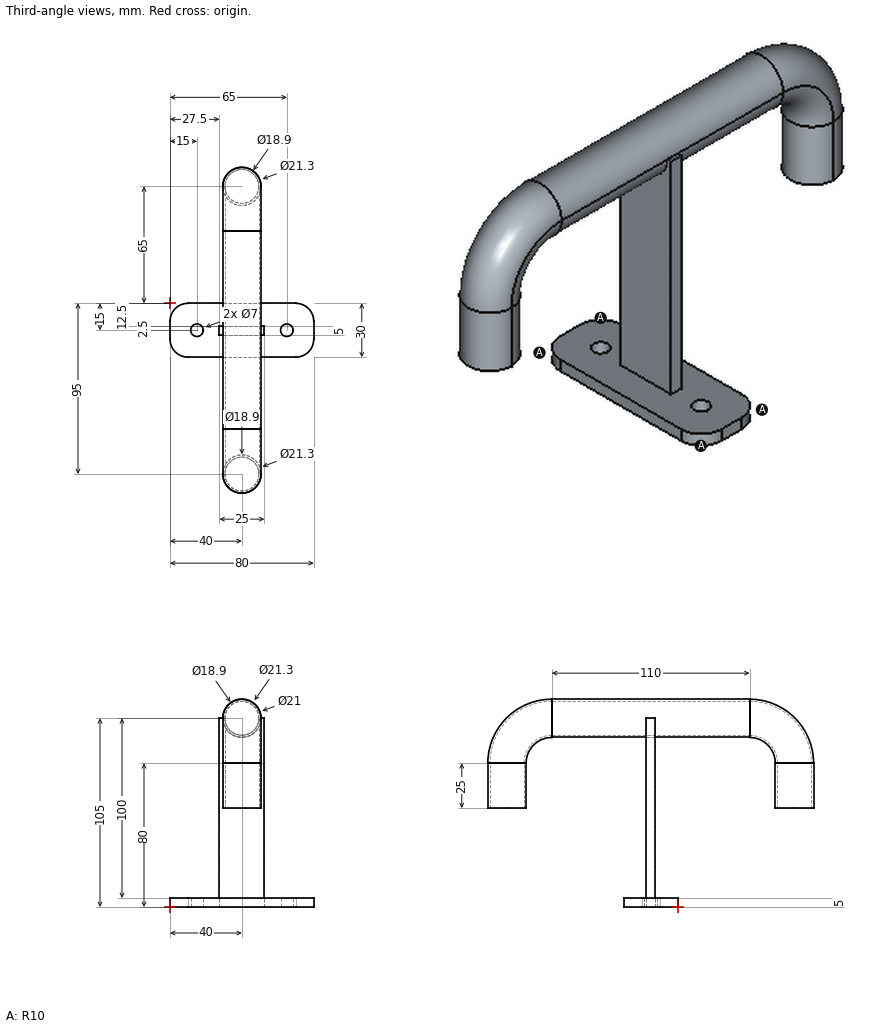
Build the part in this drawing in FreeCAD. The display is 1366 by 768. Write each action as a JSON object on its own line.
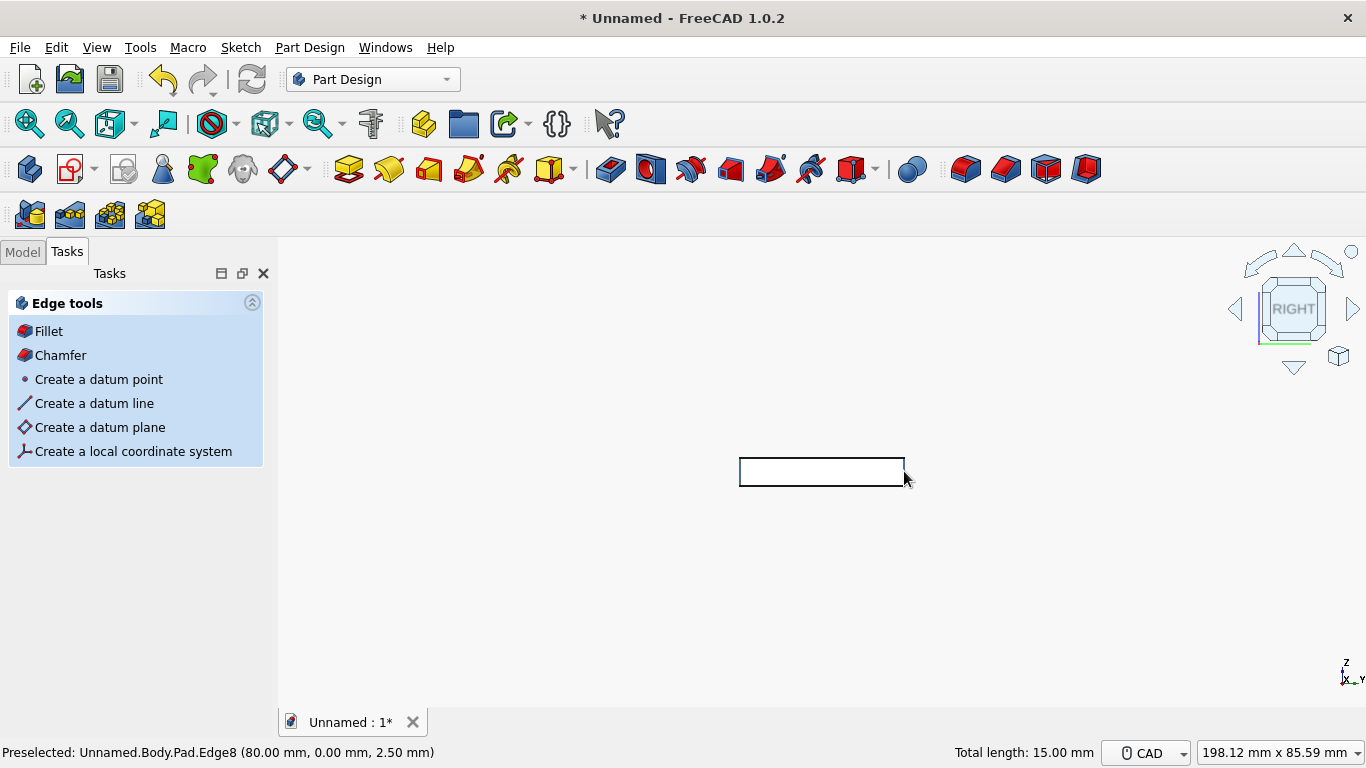
{"action": "key", "text": "5"}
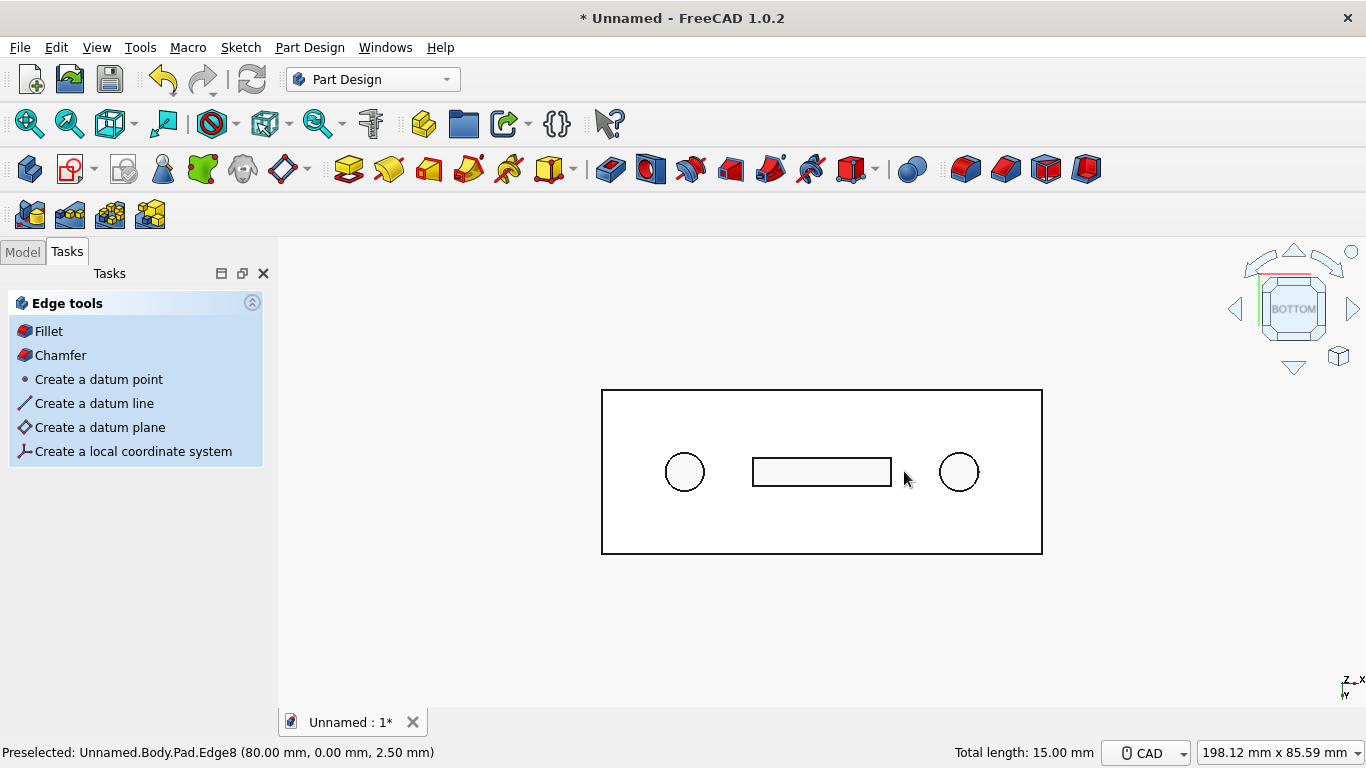
{"action": "left_click", "coordinate": [30, 124]}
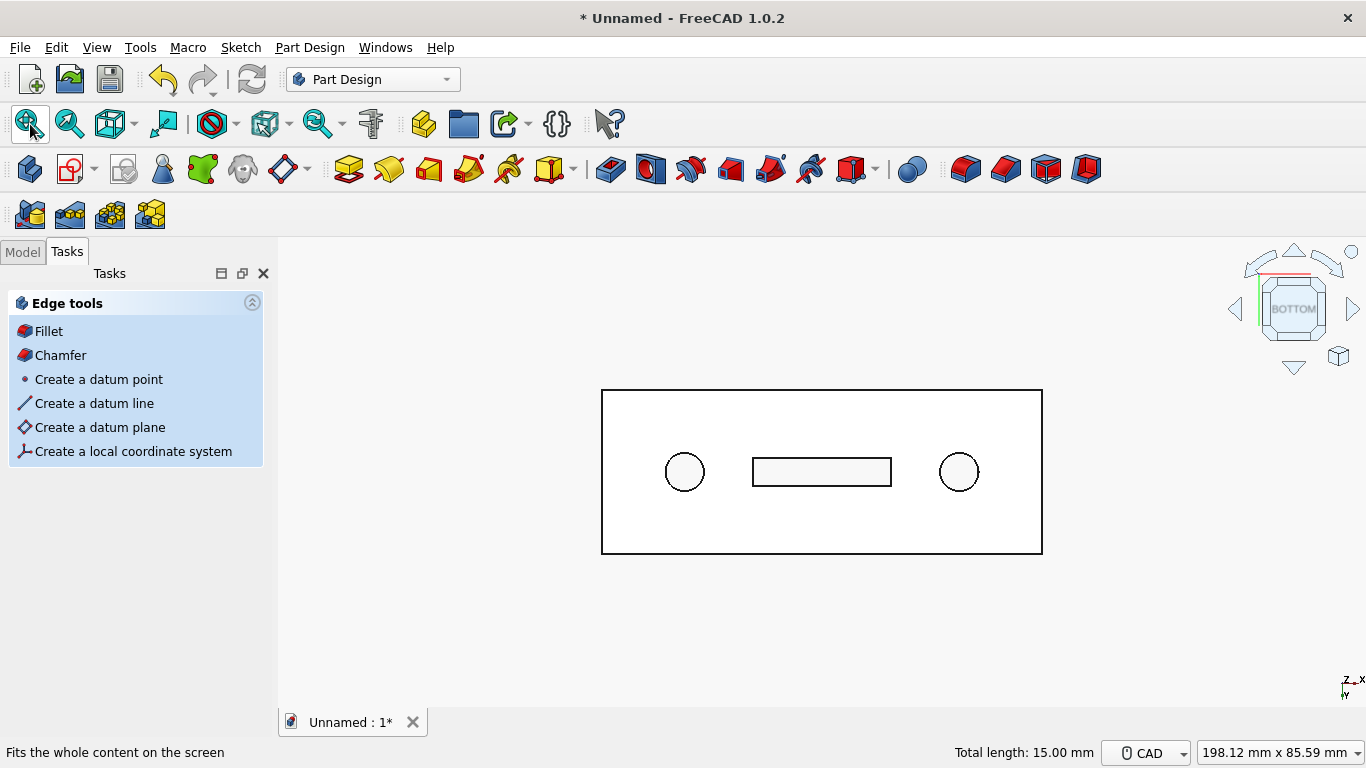
{"action": "key", "text": "4"}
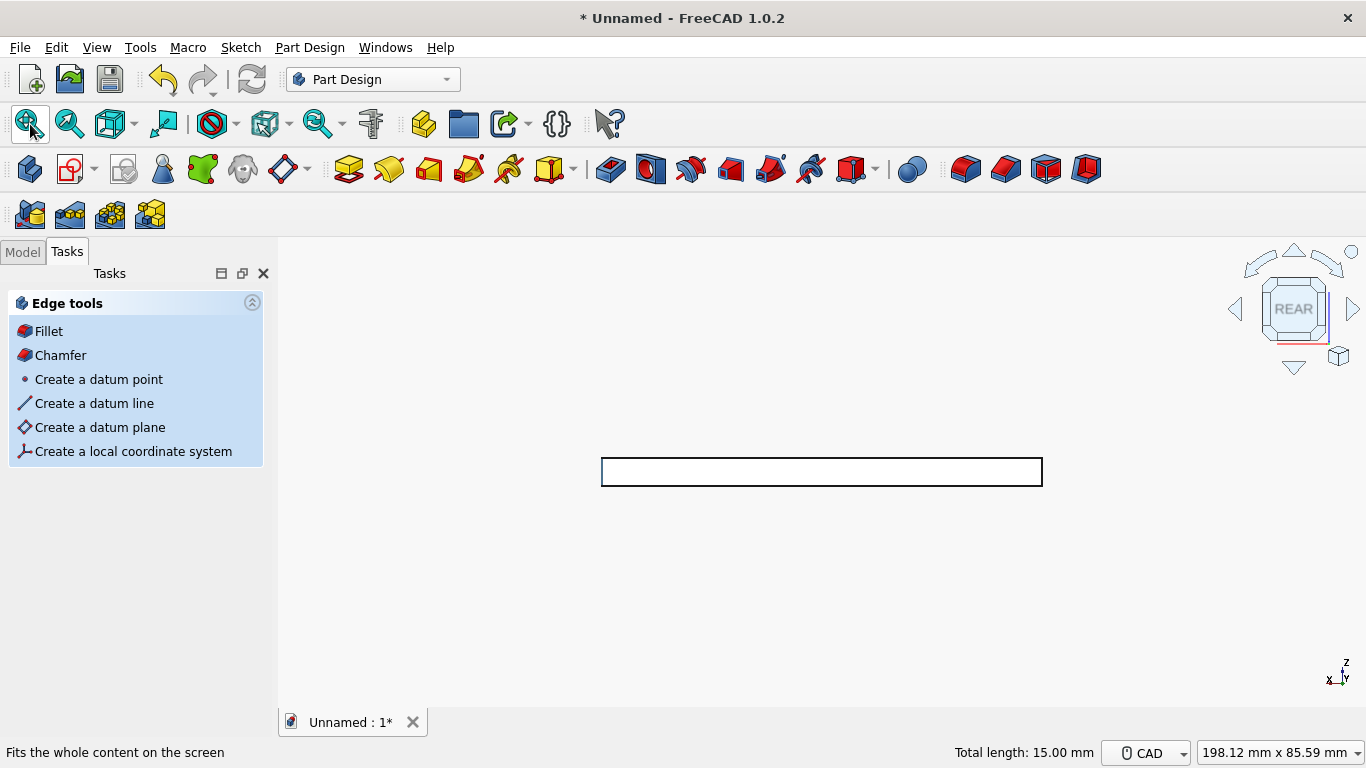
{"action": "left_click", "coordinate": [30, 124]}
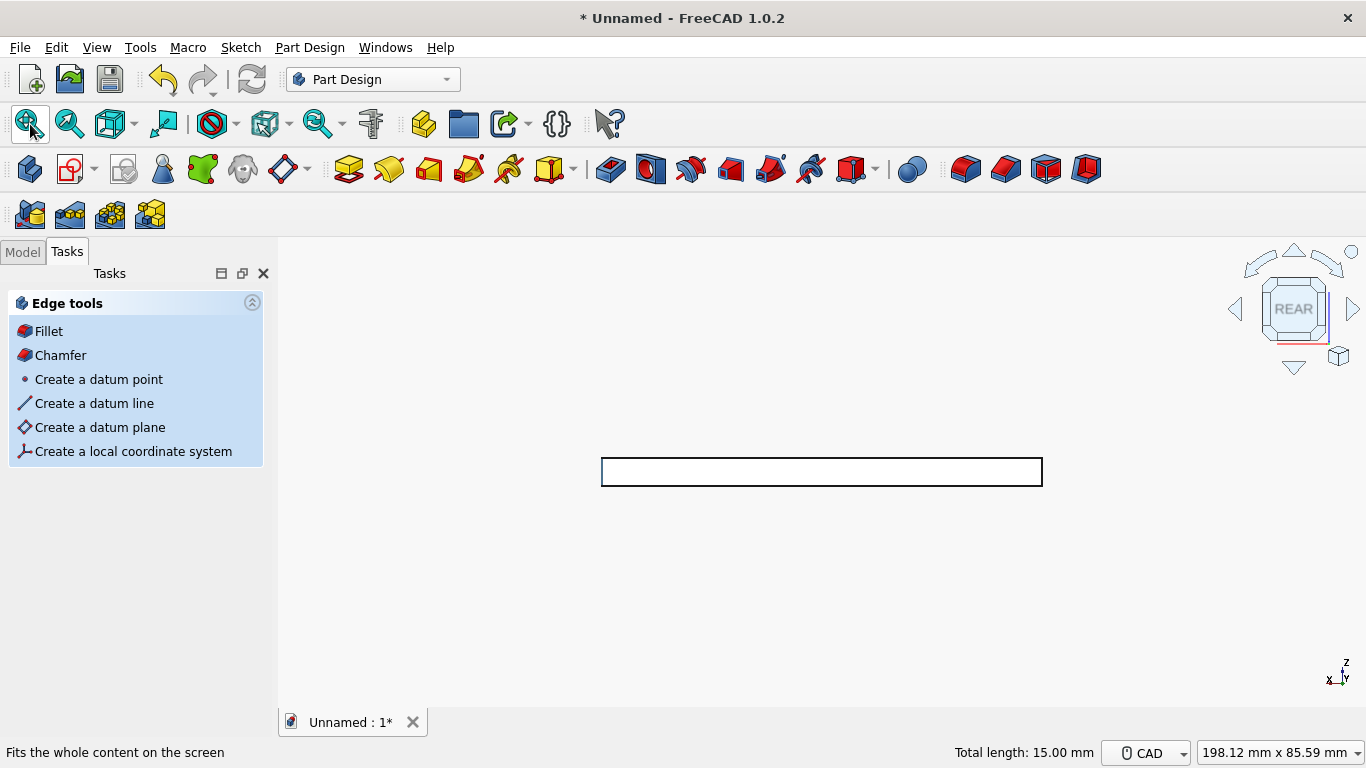
{"action": "left_click", "coordinate": [1042, 471], "text": "ctrl"}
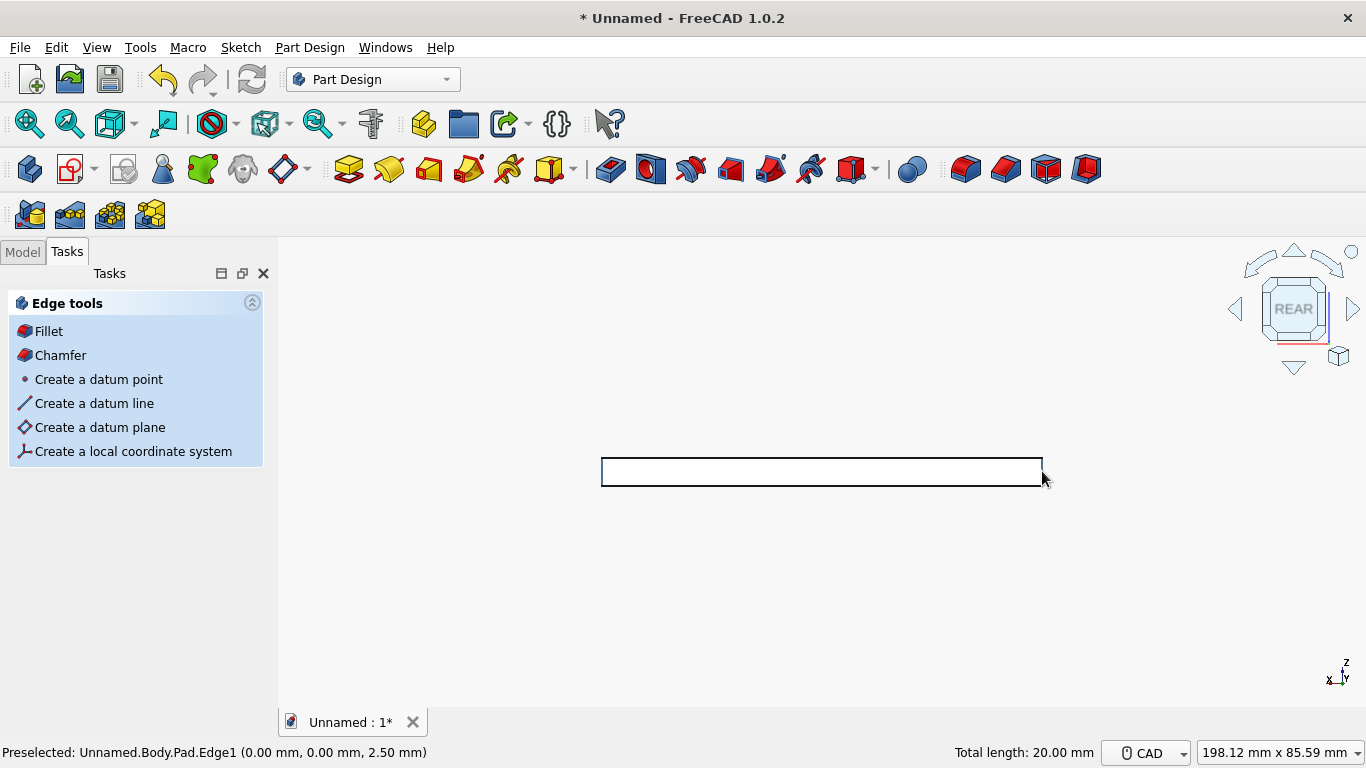
{"action": "left_click", "coordinate": [966, 170]}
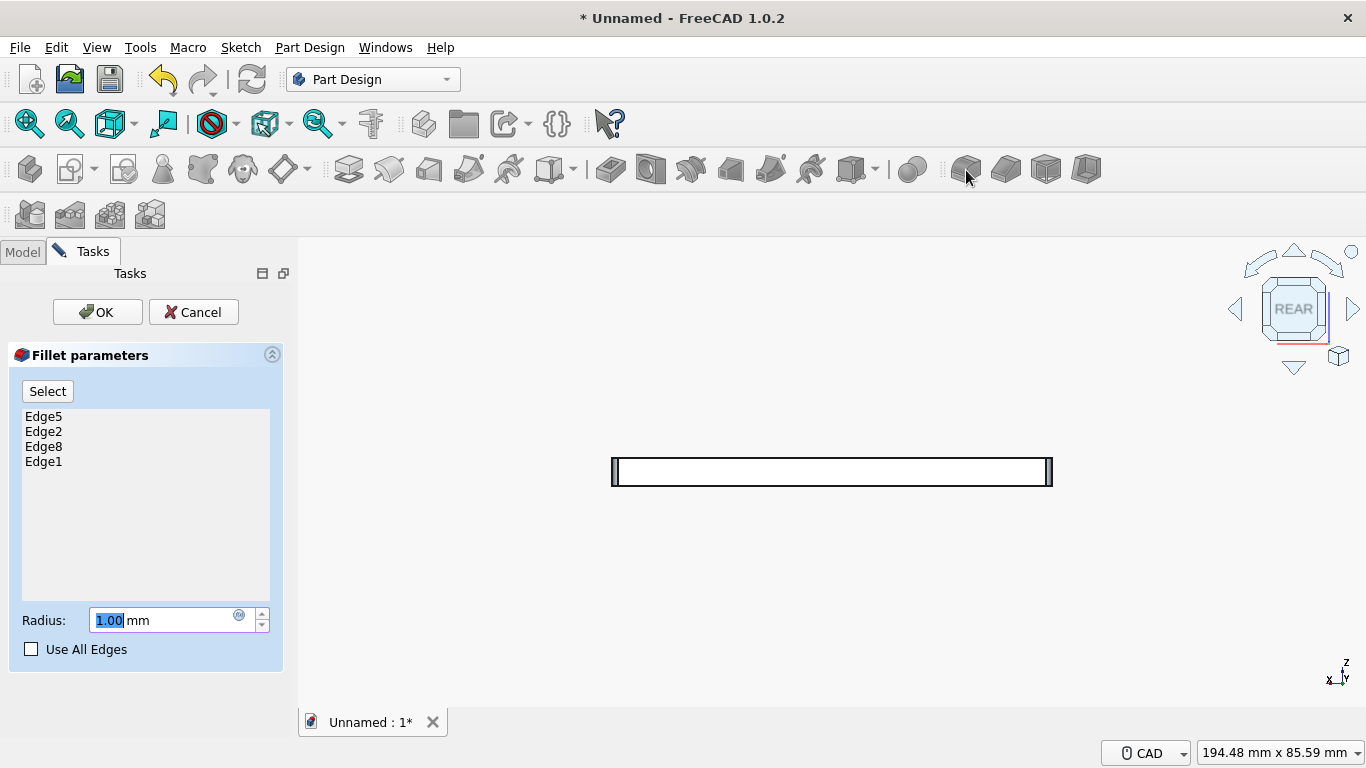
{"action": "type", "text": "10"}
{"action": "key", "text": "Tab"}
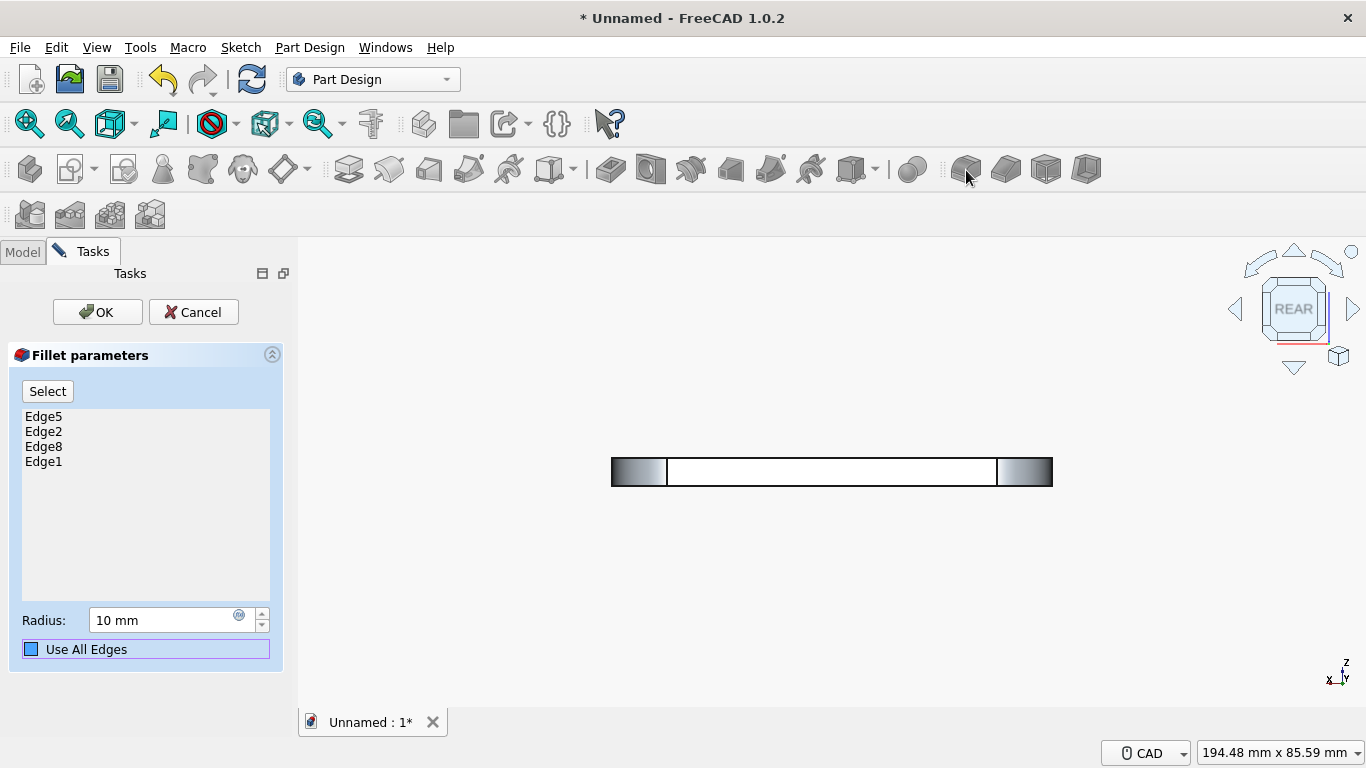
{"action": "left_click", "coordinate": [98, 312]}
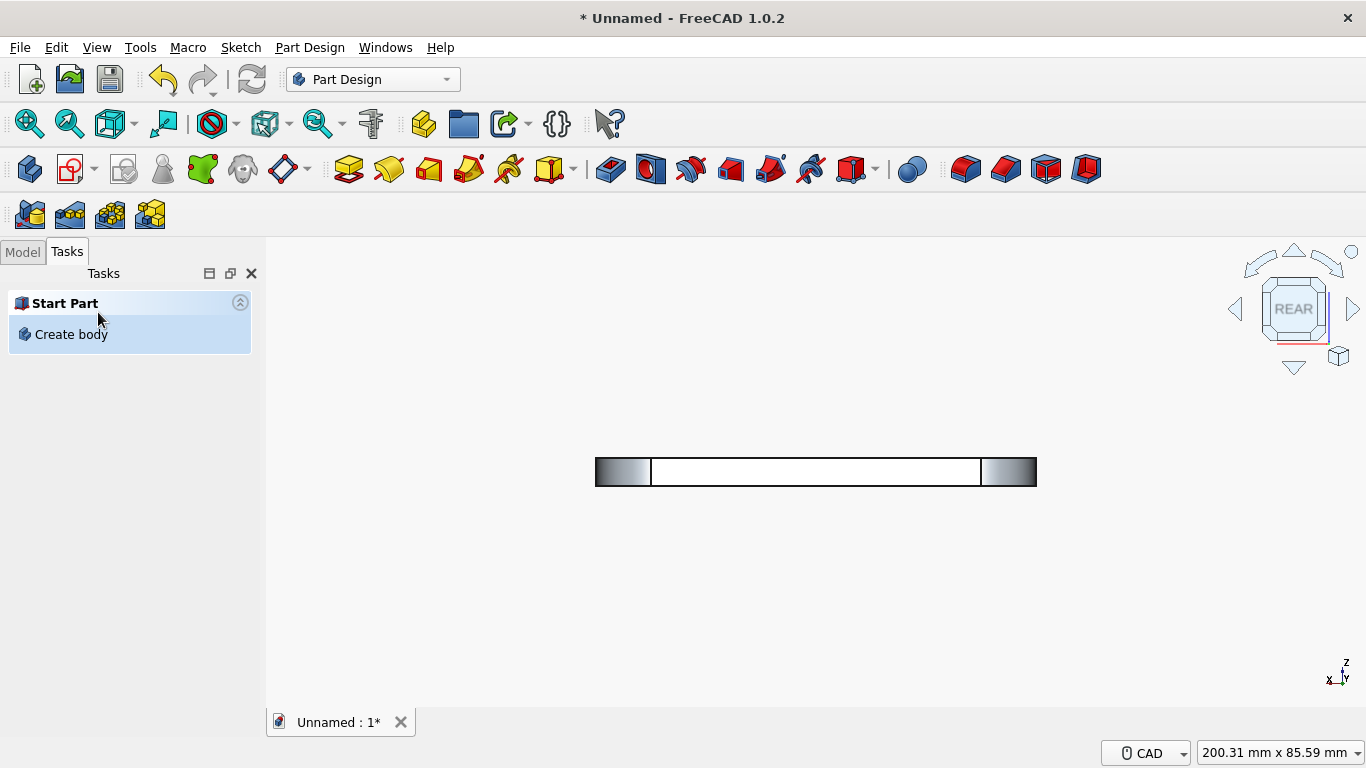
{"action": "left_click", "coordinate": [30, 124]}